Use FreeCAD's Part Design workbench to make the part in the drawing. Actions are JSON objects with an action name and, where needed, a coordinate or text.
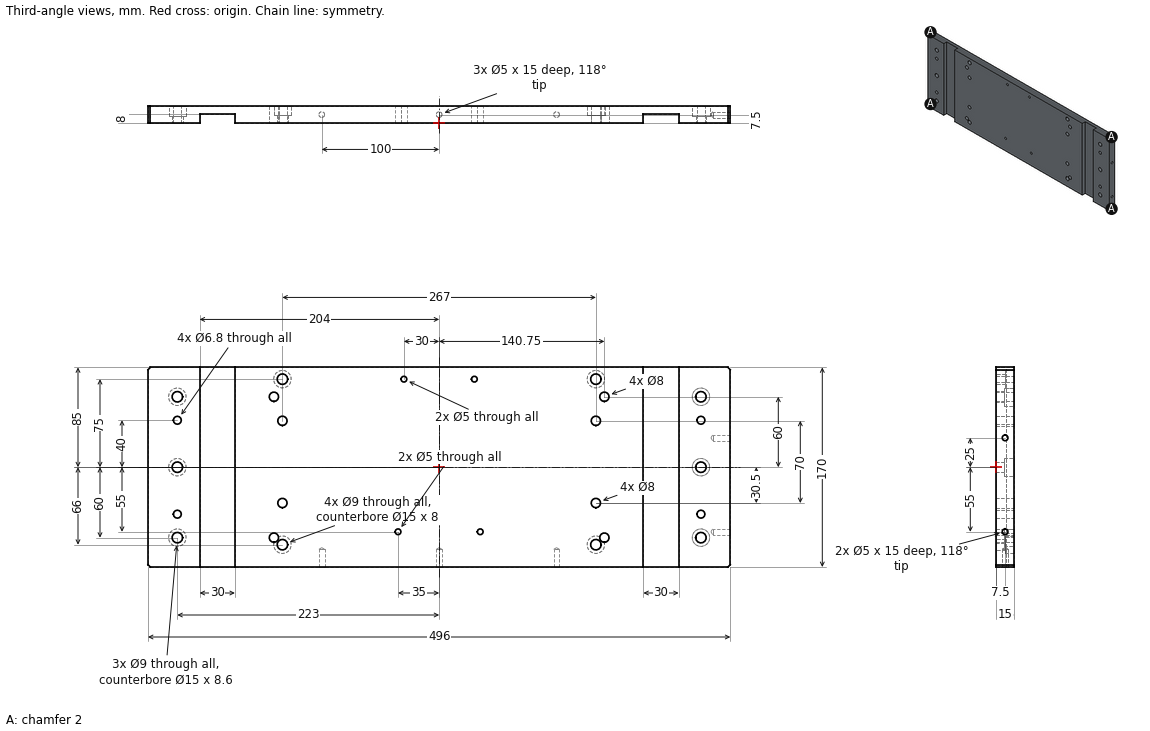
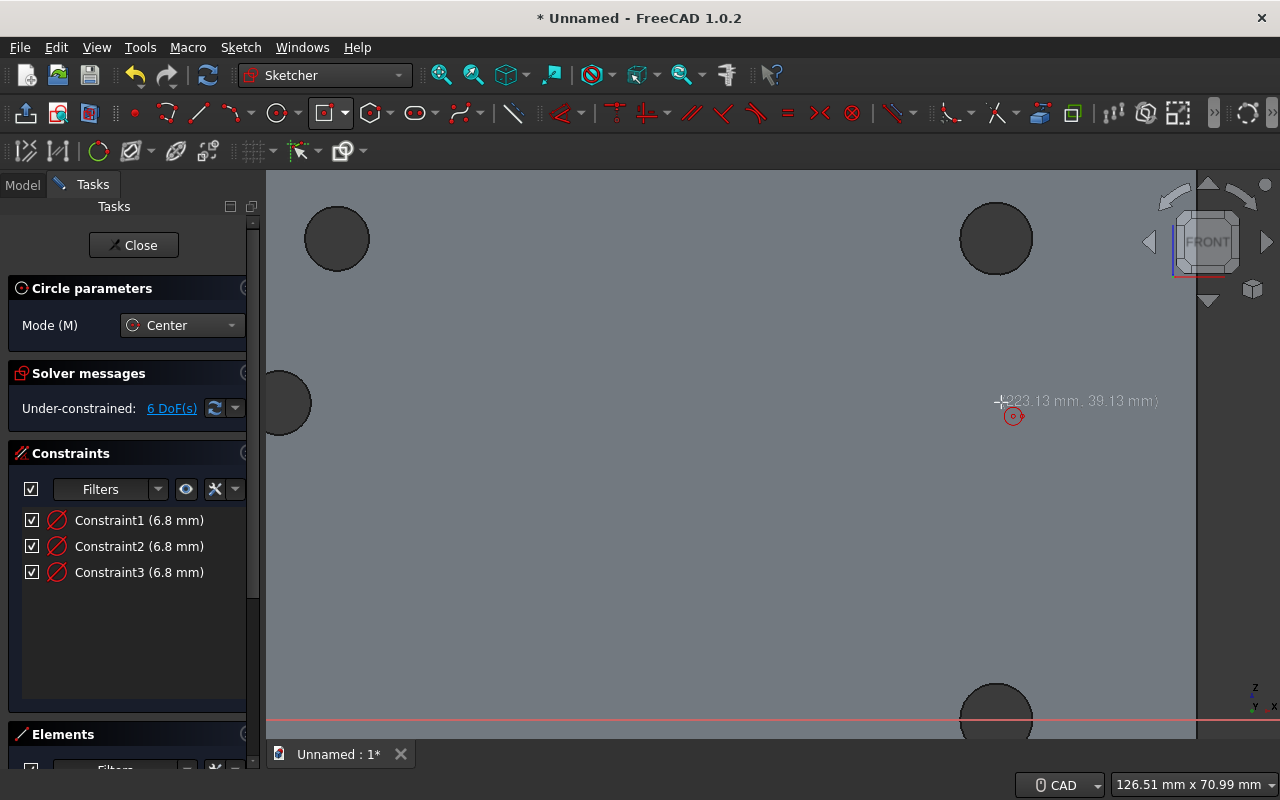
{"action": "scroll", "coordinate": [1001, 402], "scroll_direction": "down", "scroll_amount": 9}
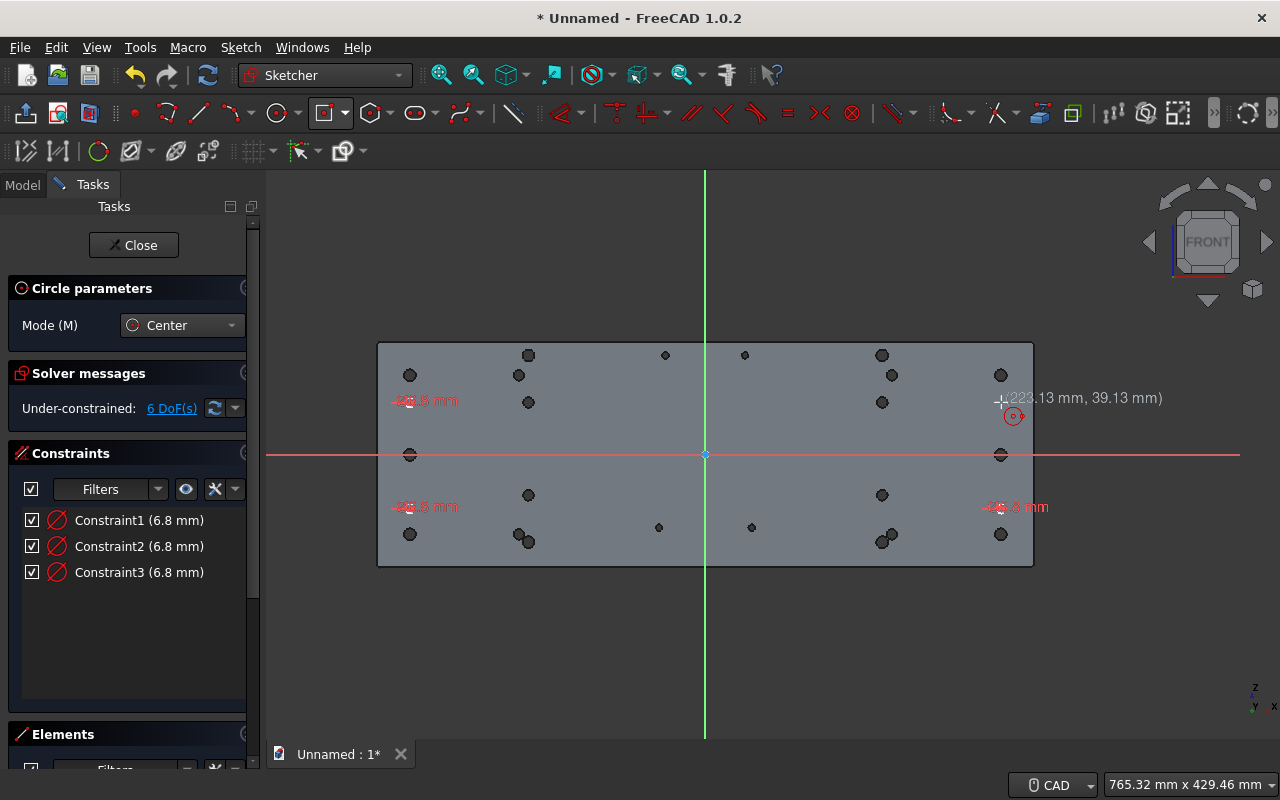
{"action": "left_click", "coordinate": [1001, 402]}
{"action": "mouse_move", "coordinate": [1004, 399]}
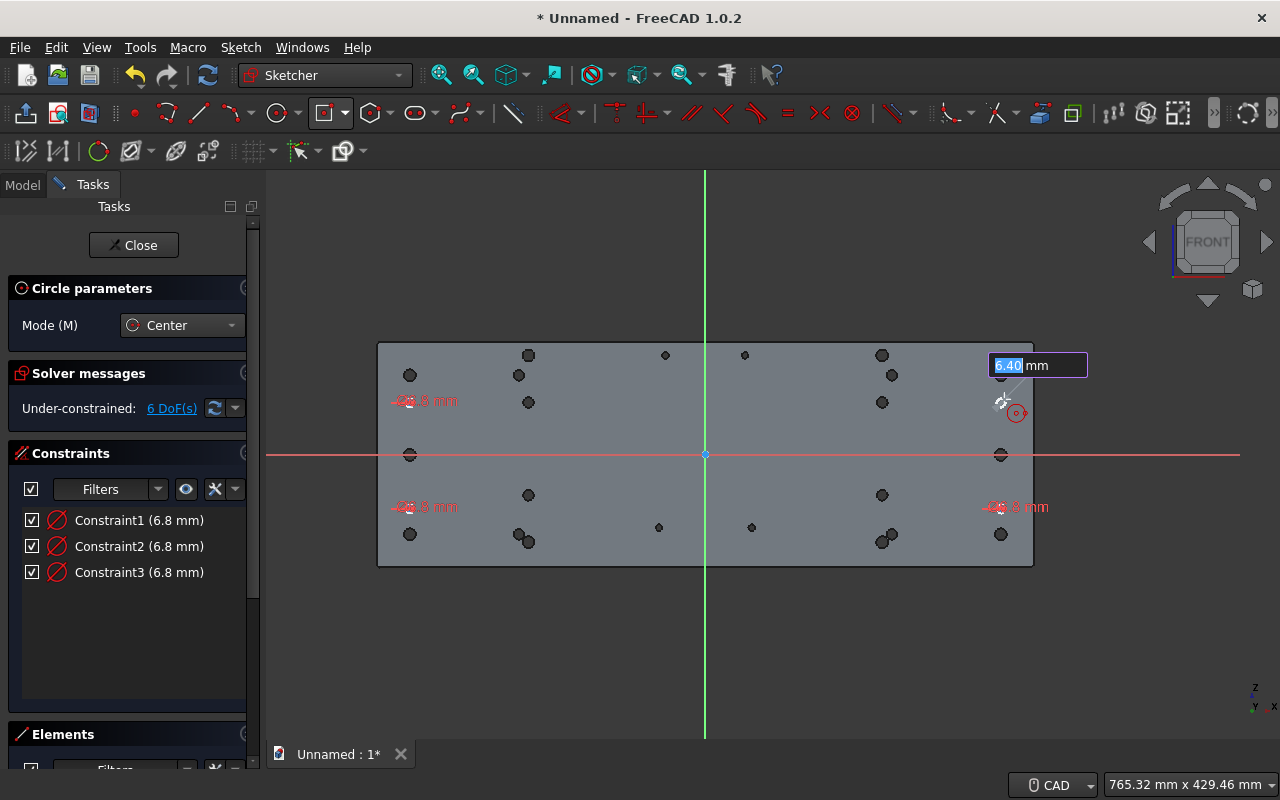
{"action": "type", "text": "6.8"}
{"action": "key", "text": "Return"}
{"action": "key", "text": "Escape"}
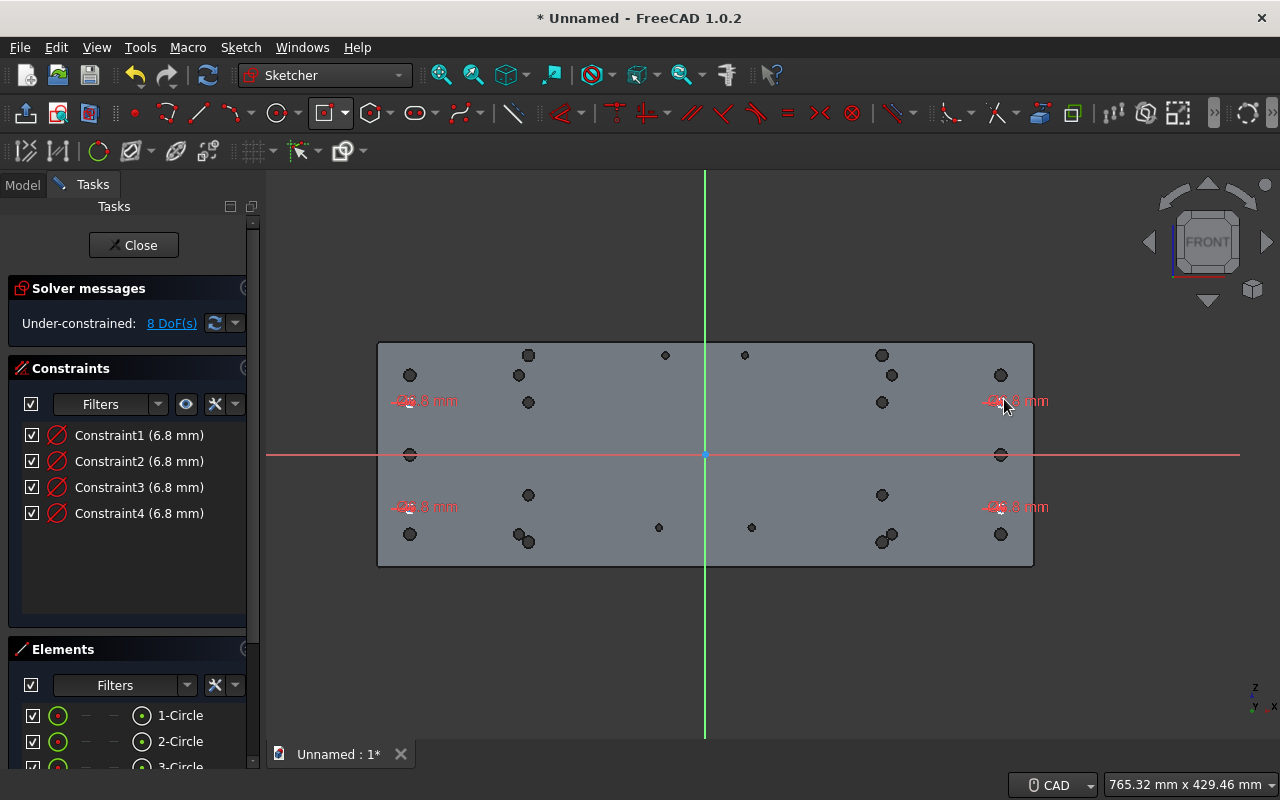
{"action": "left_click", "coordinate": [410, 403]}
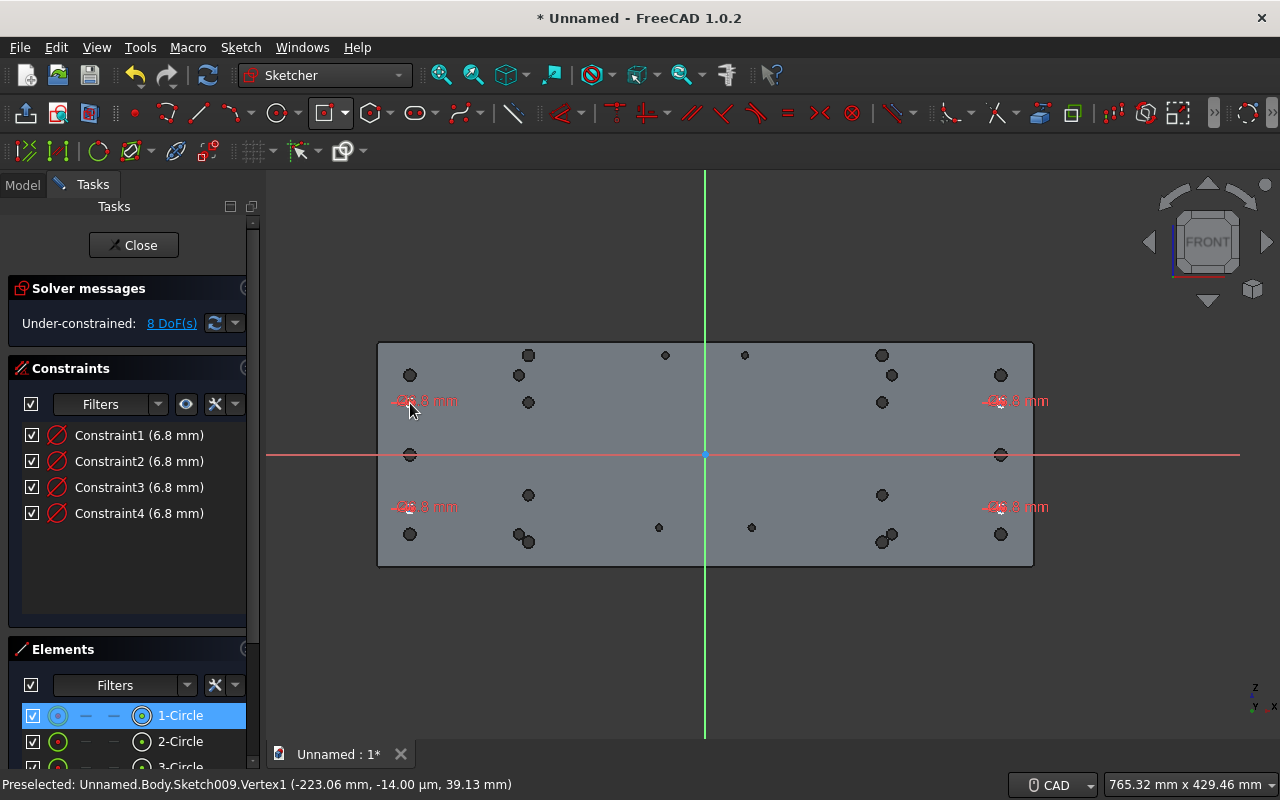
{"action": "left_click", "coordinate": [410, 509]}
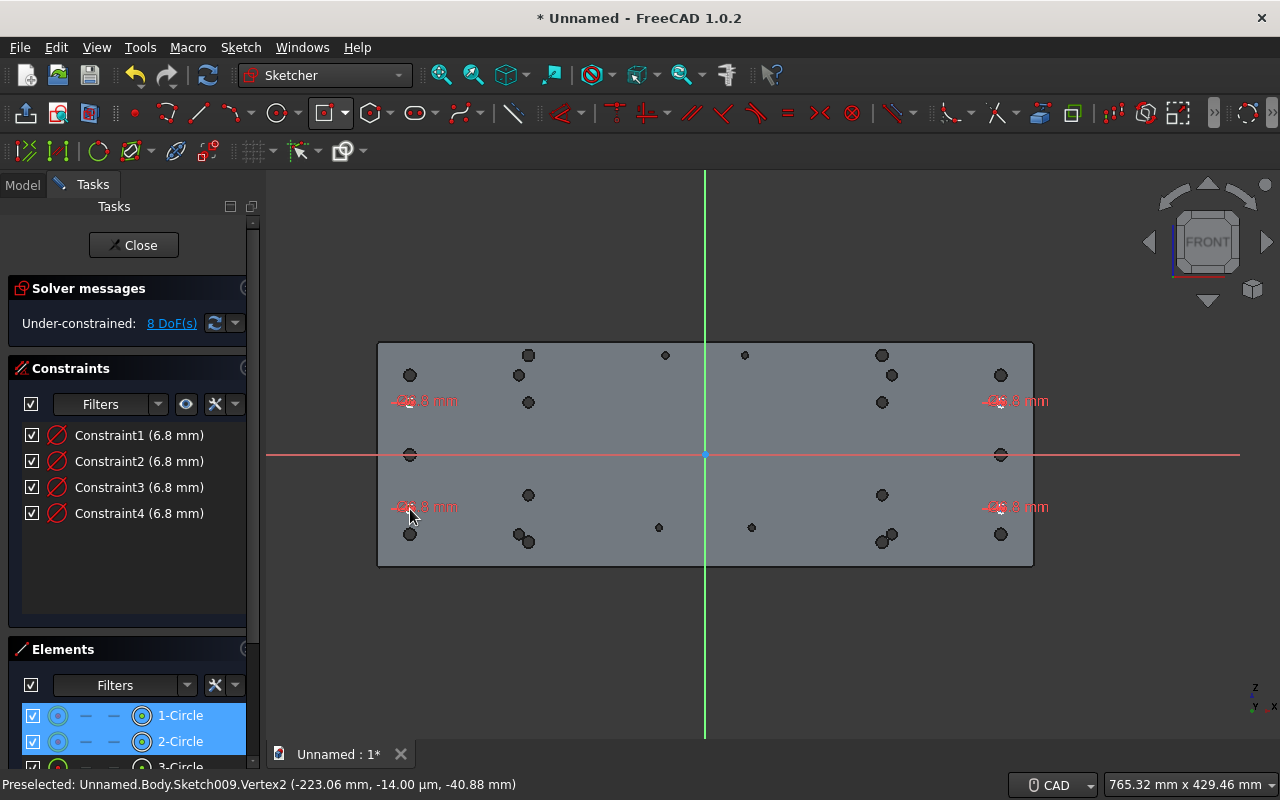
{"action": "left_click", "coordinate": [353, 455]}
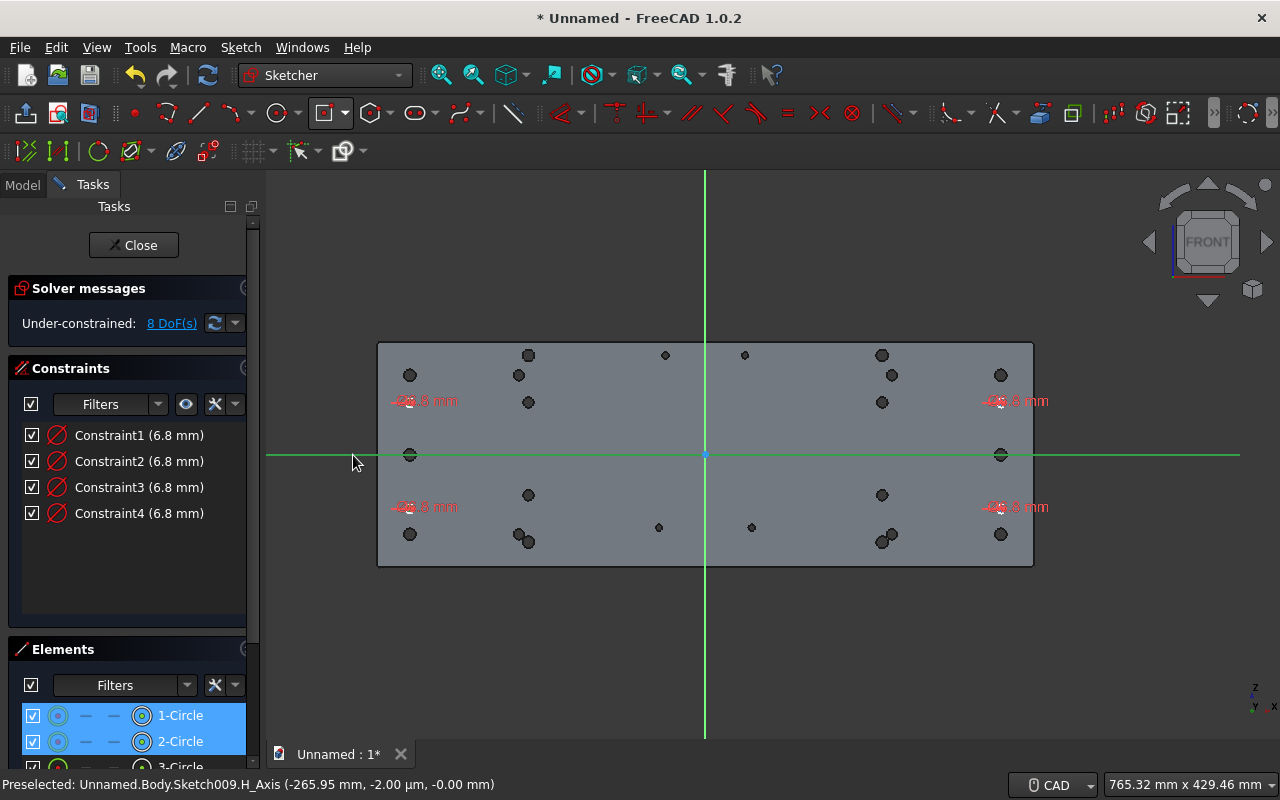
{"action": "left_click", "coordinate": [820, 114]}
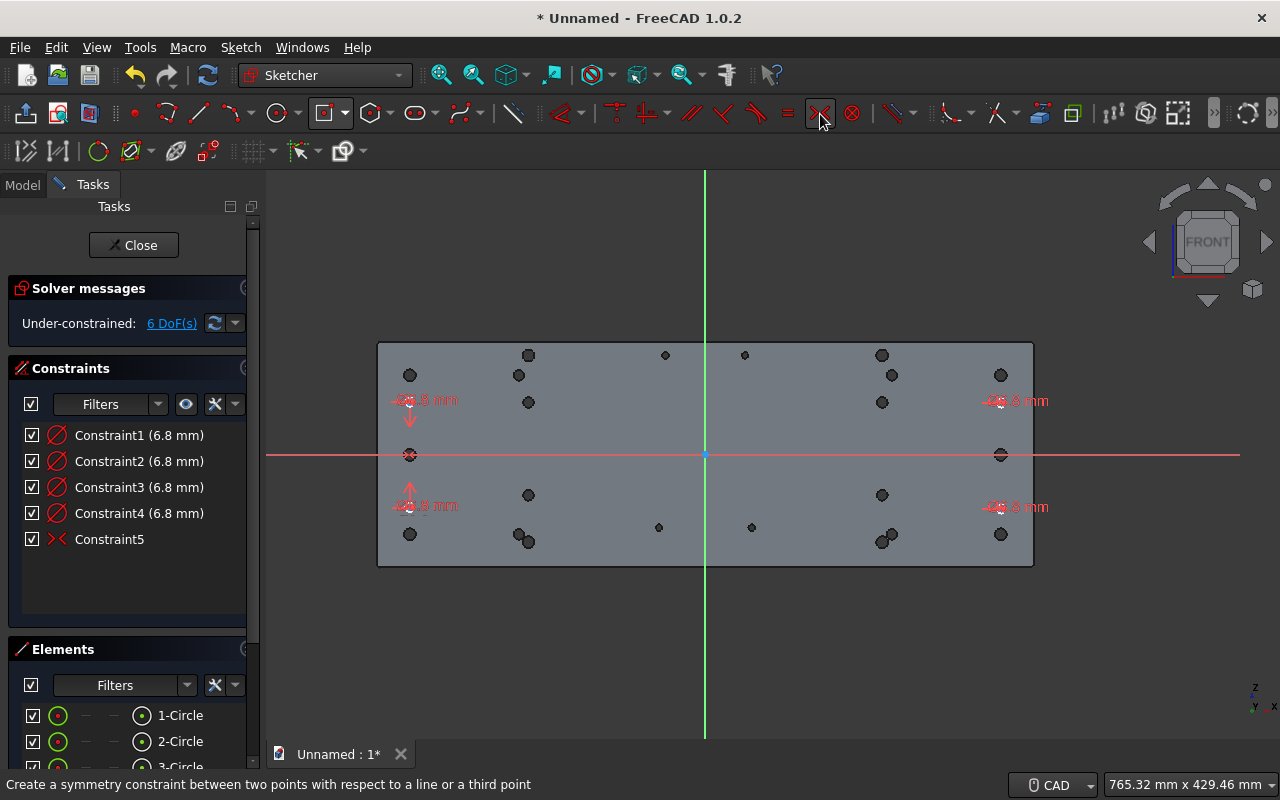
{"action": "left_click", "coordinate": [410, 508]}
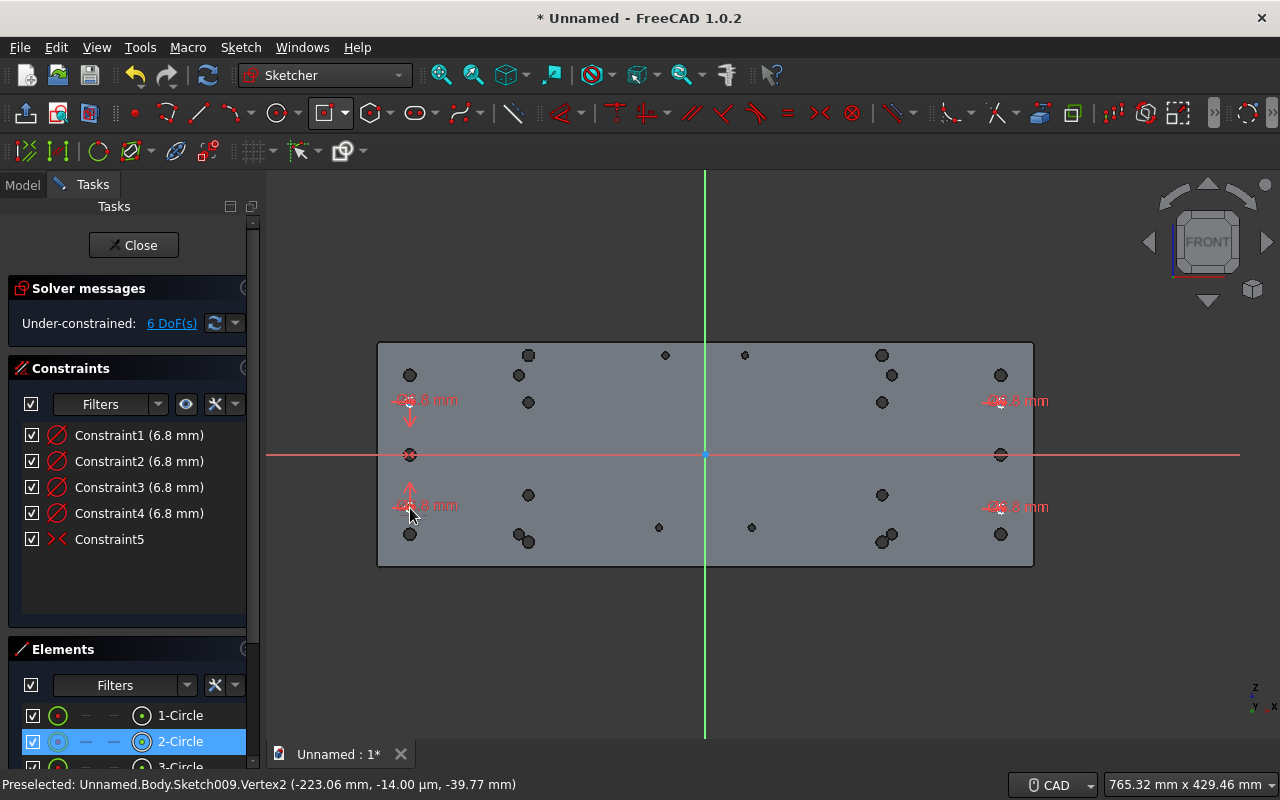
{"action": "left_click", "coordinate": [1001, 509]}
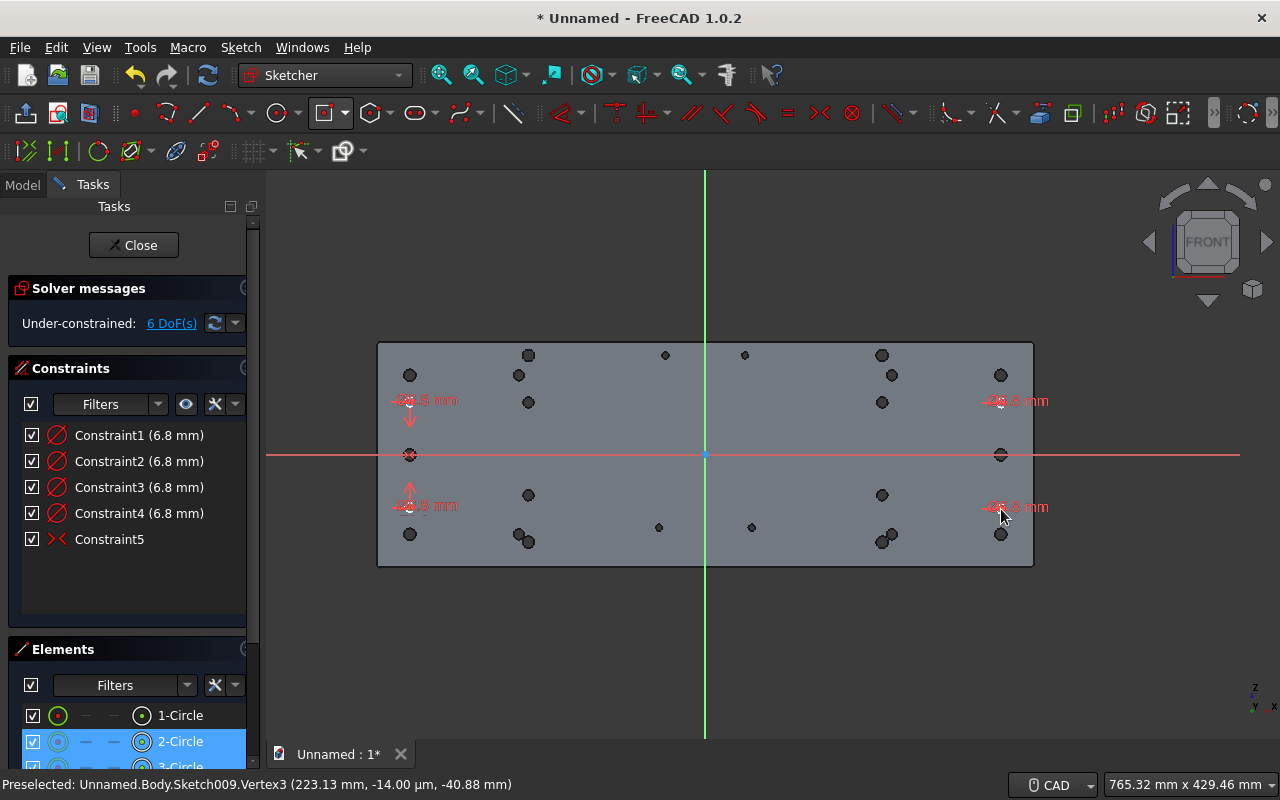
{"action": "left_click", "coordinate": [705, 674]}